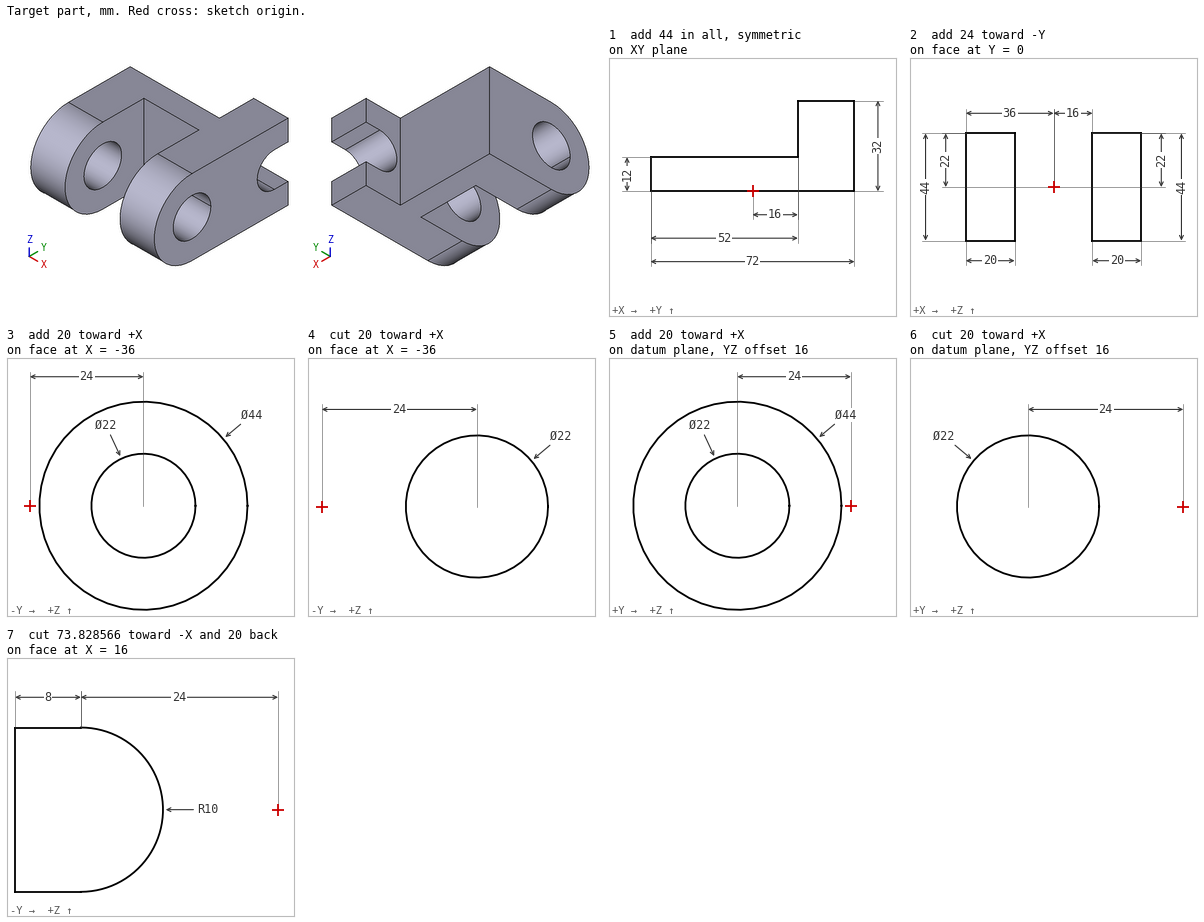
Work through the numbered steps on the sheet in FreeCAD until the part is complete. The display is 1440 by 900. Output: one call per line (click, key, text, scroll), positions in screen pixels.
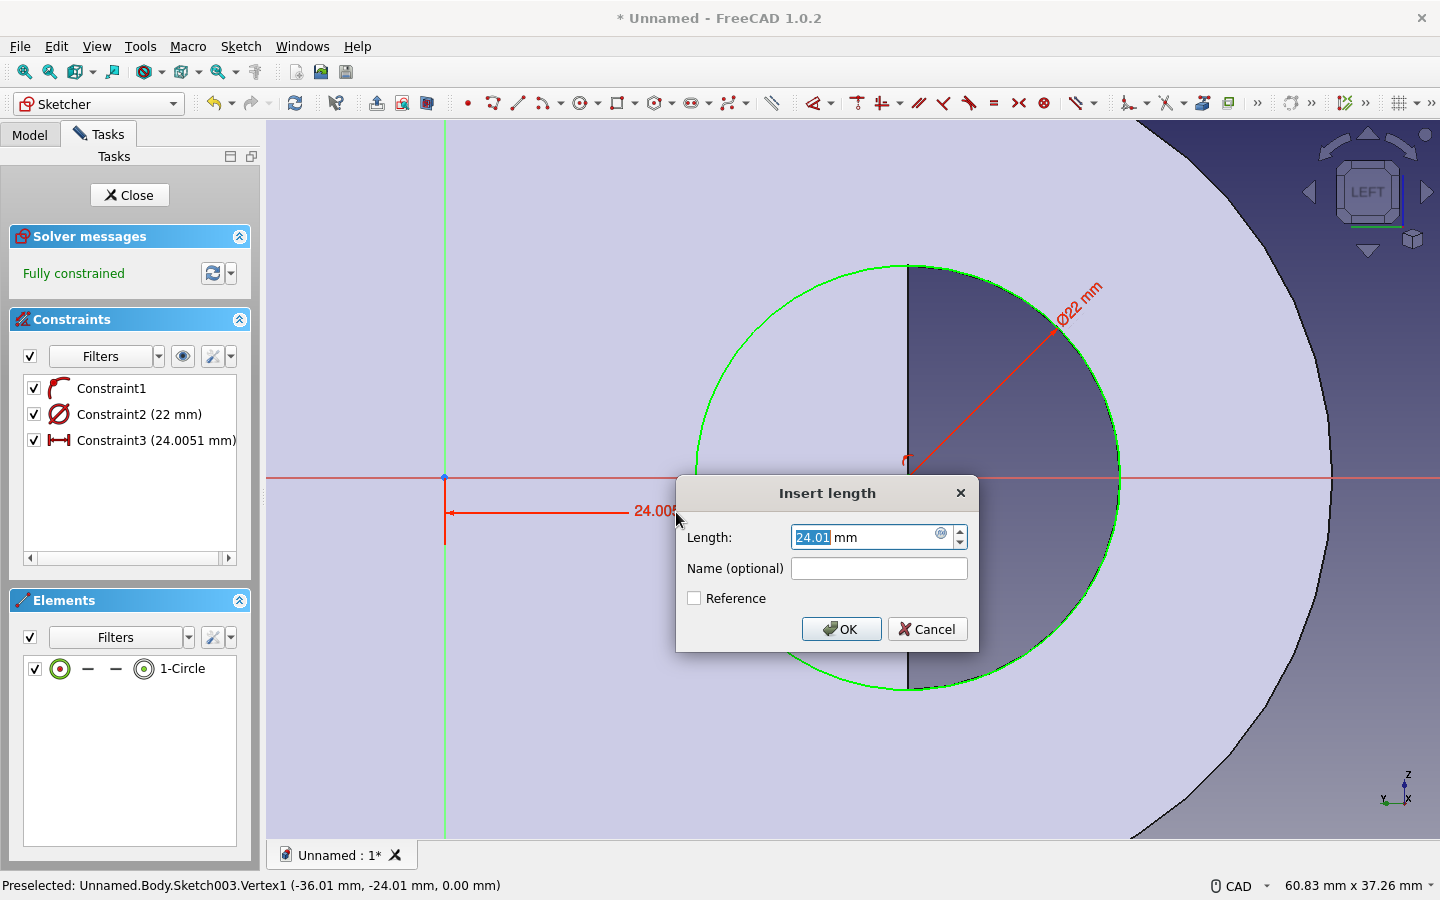
text(24)
key(Return)
key(Escape)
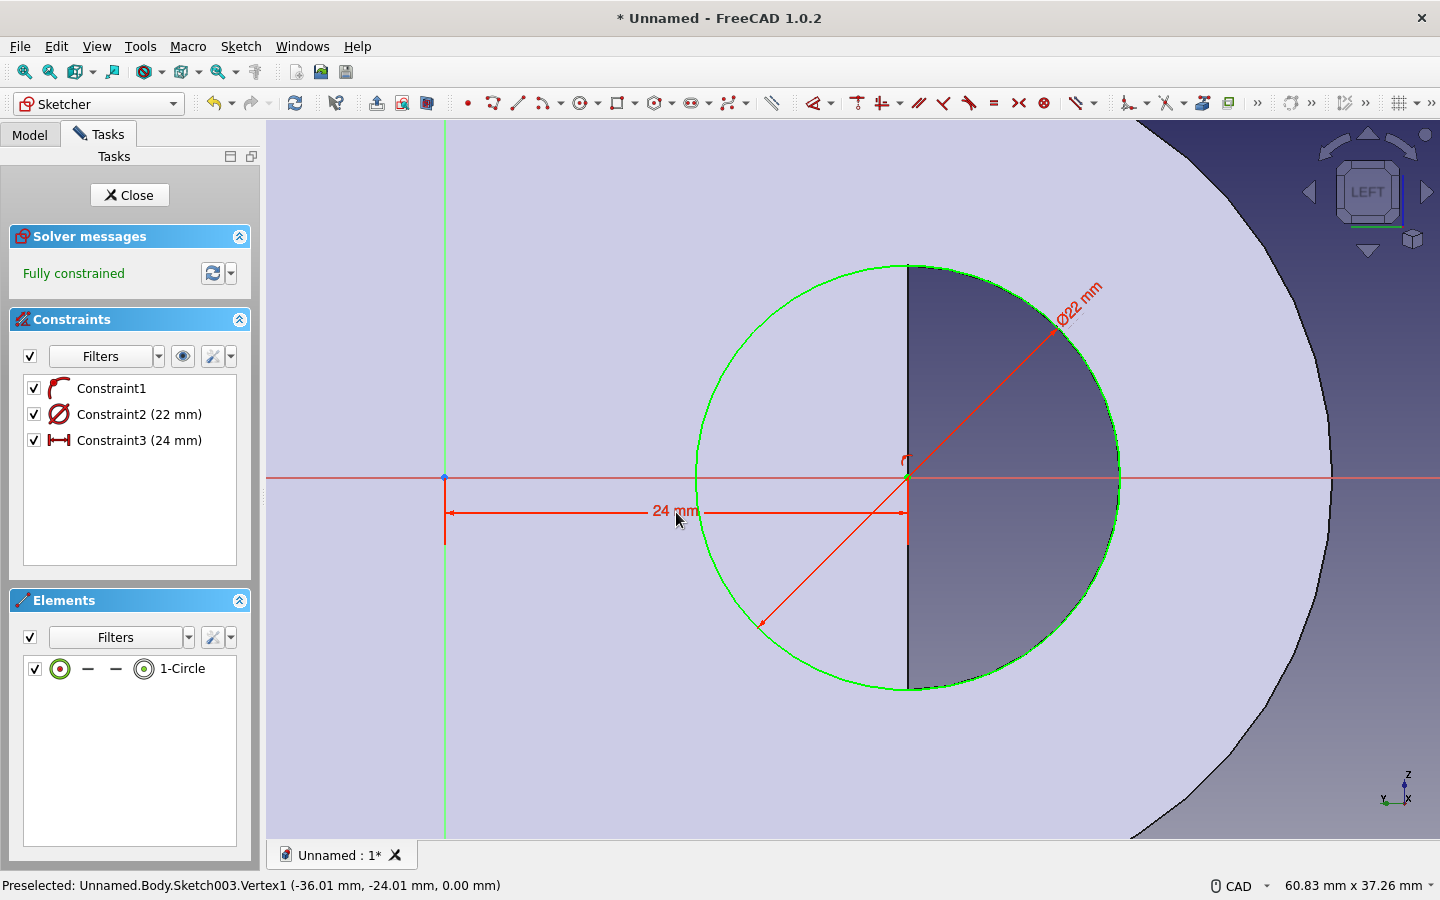
click(130, 195)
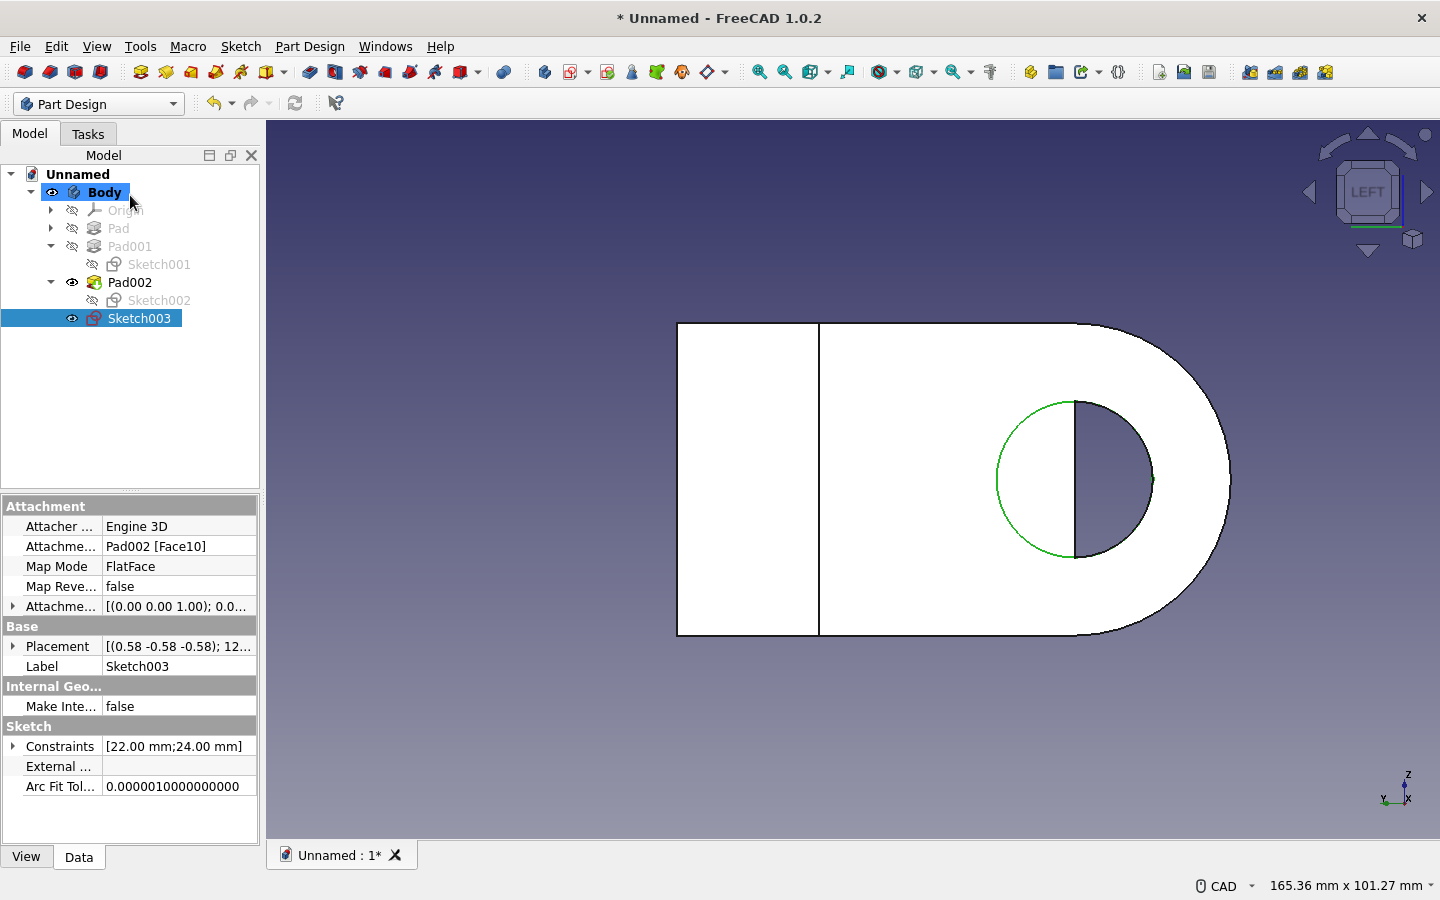
click(310, 72)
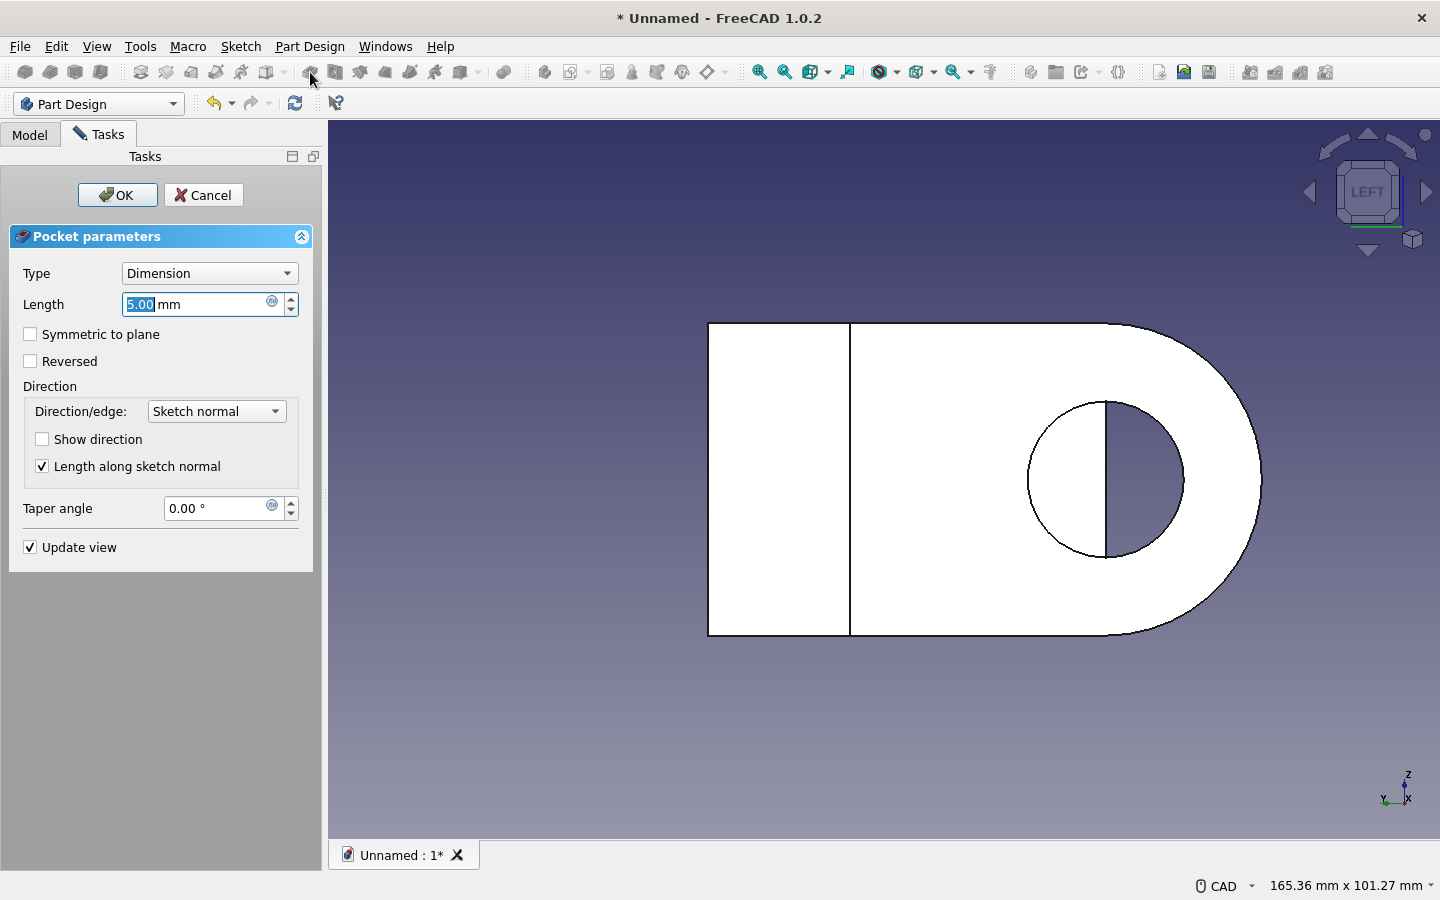
text(20)
key(Tab)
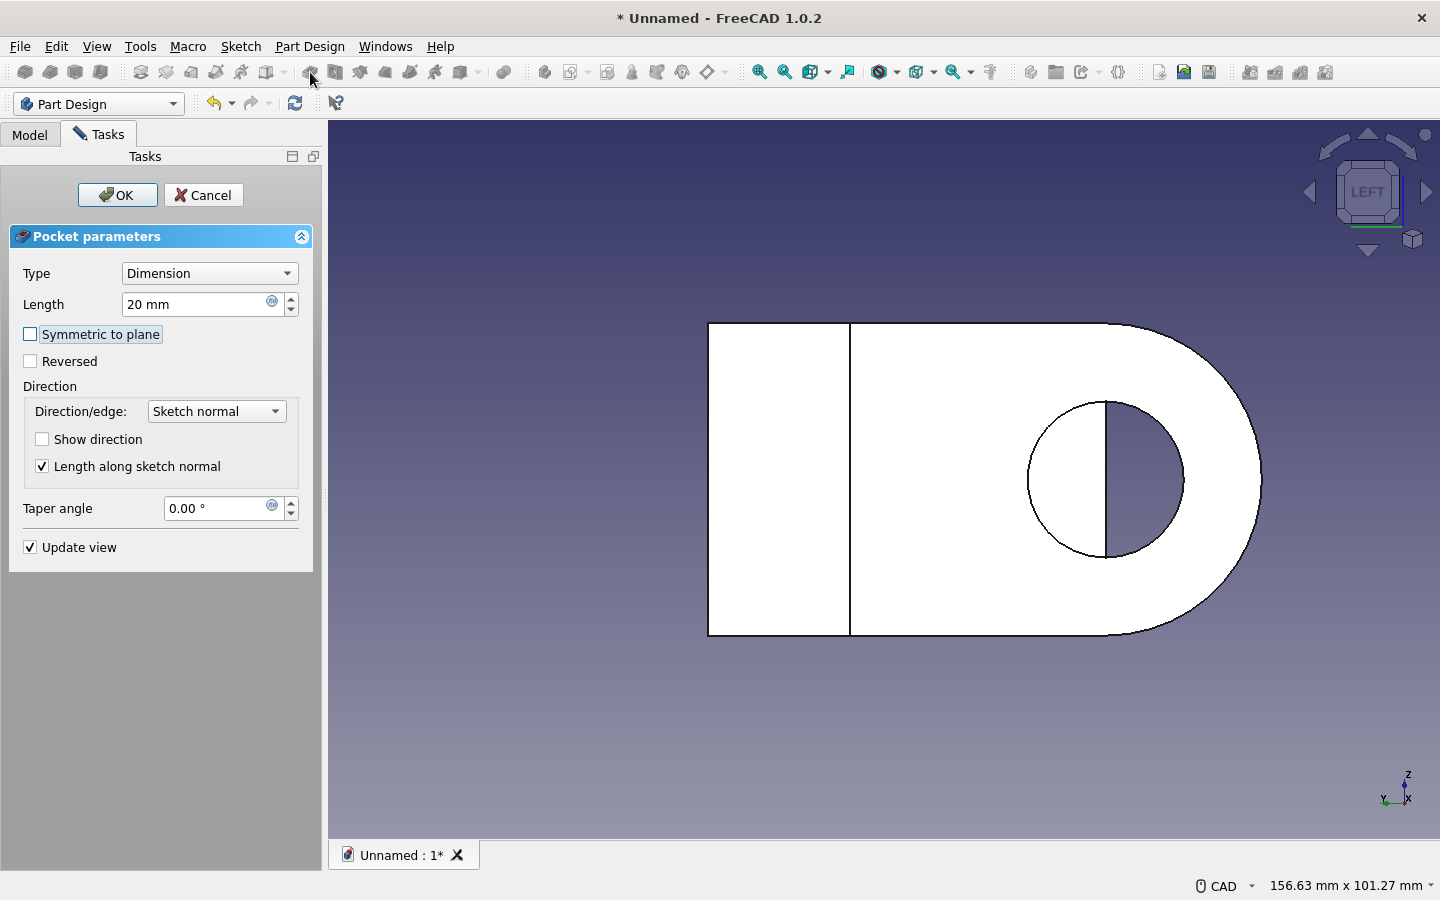
click(118, 195)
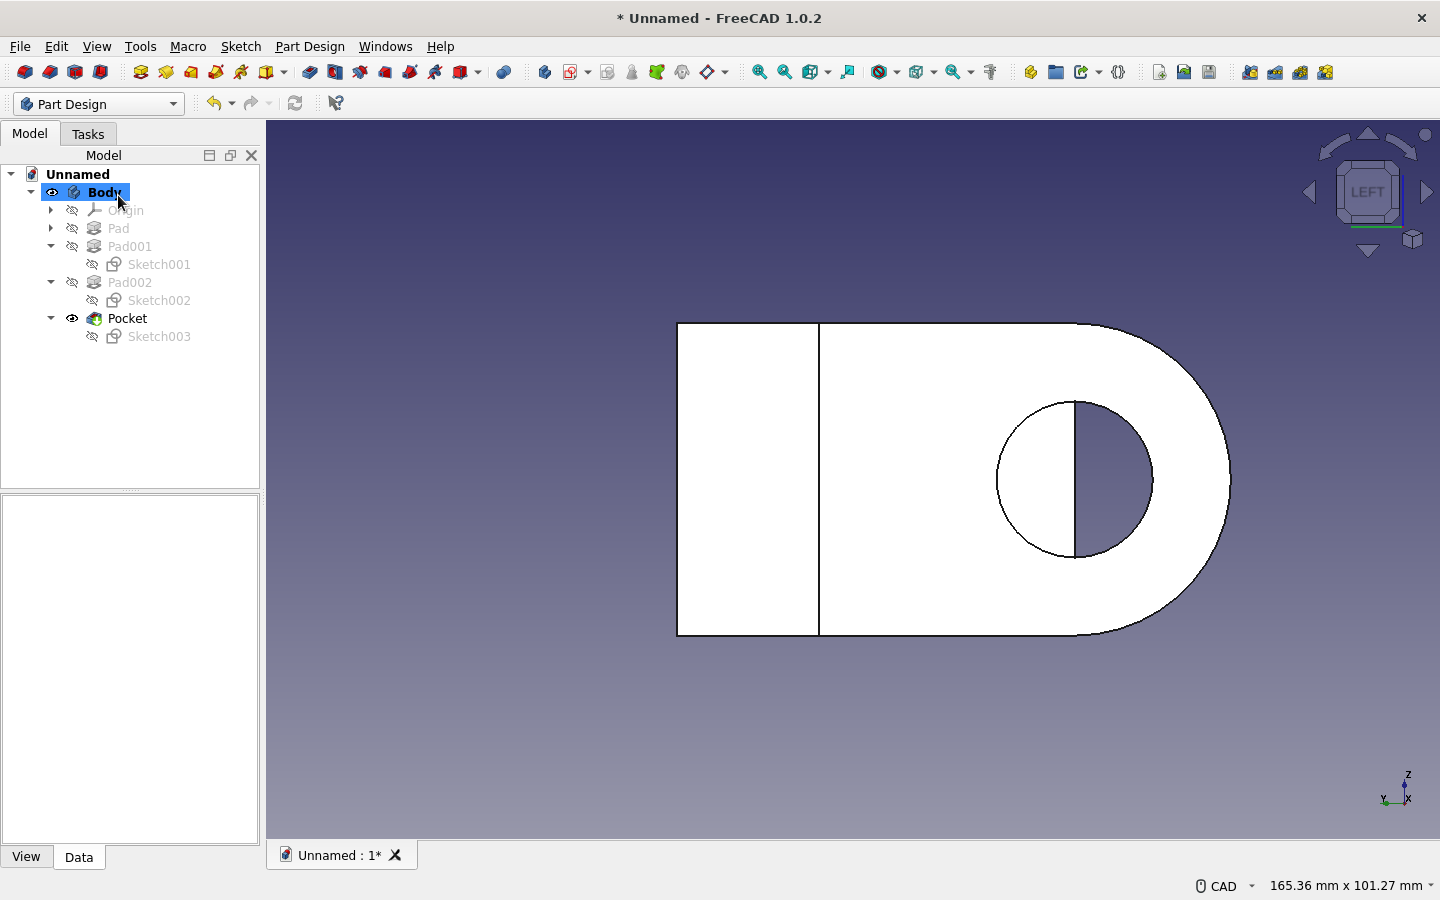
key(2)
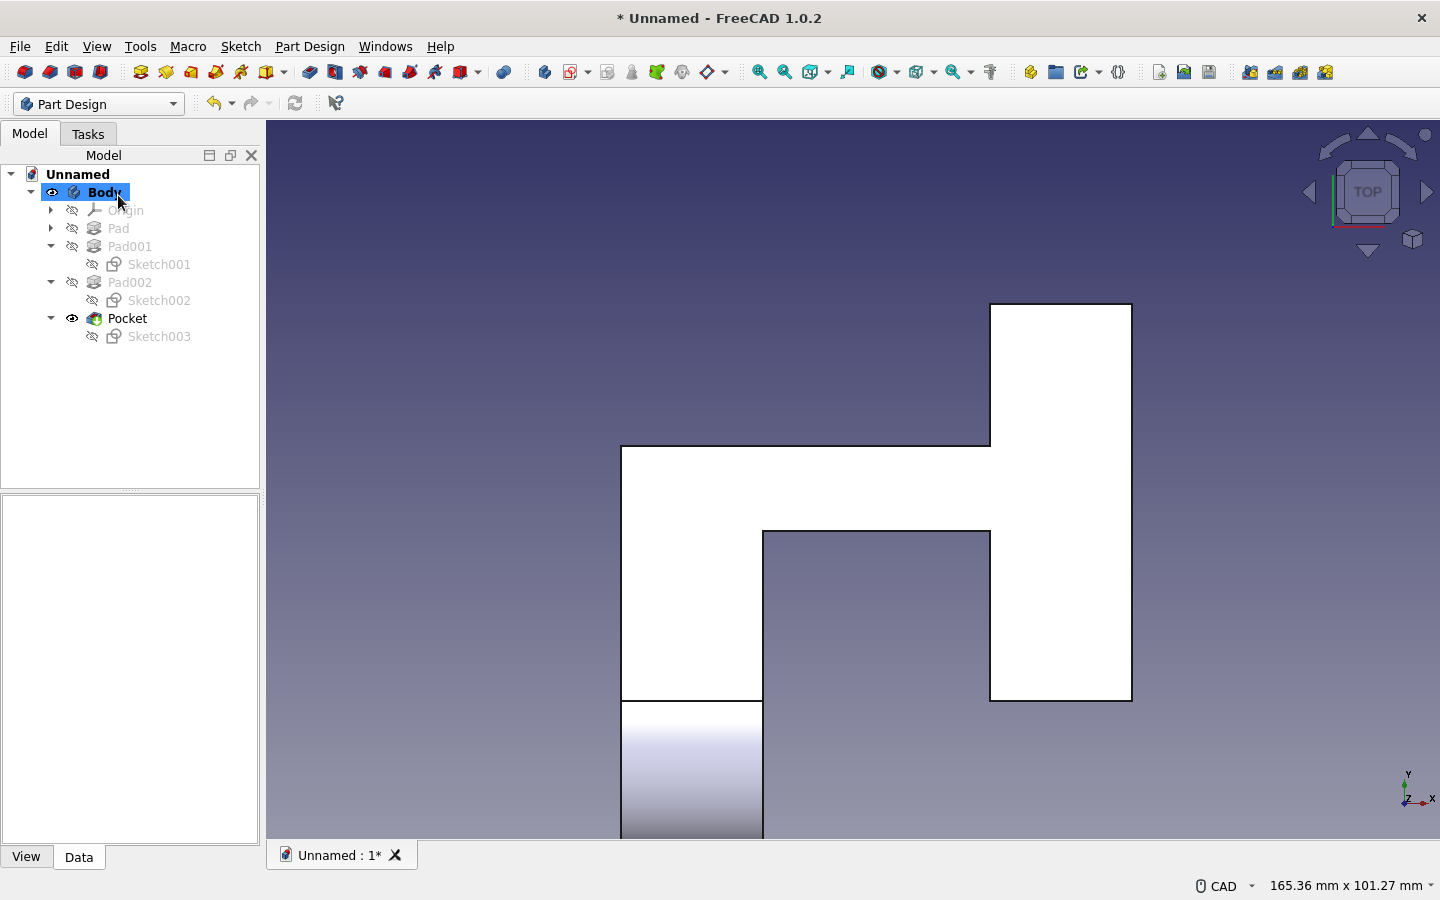
click(760, 72)